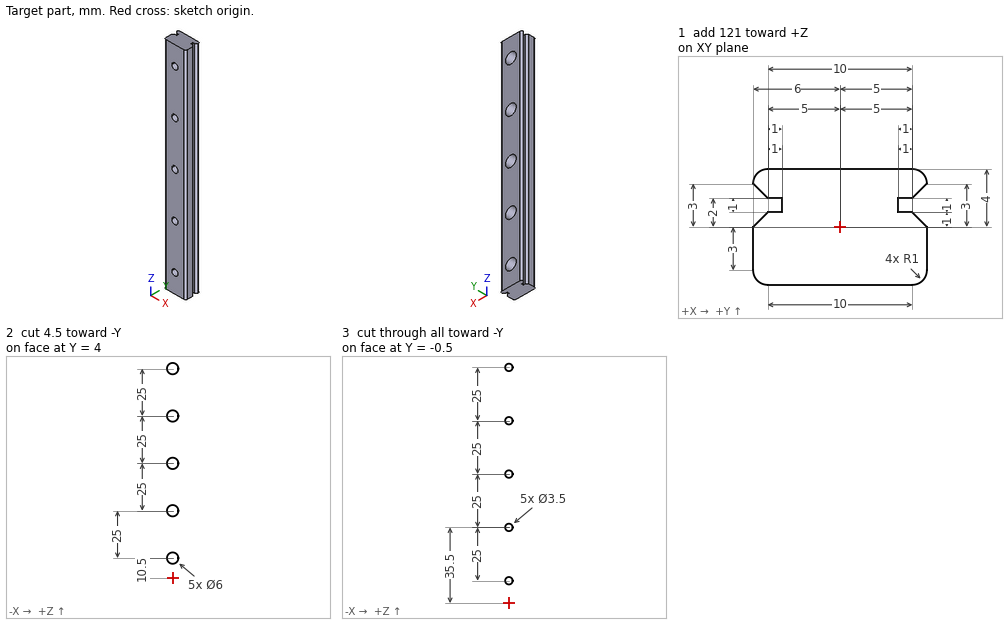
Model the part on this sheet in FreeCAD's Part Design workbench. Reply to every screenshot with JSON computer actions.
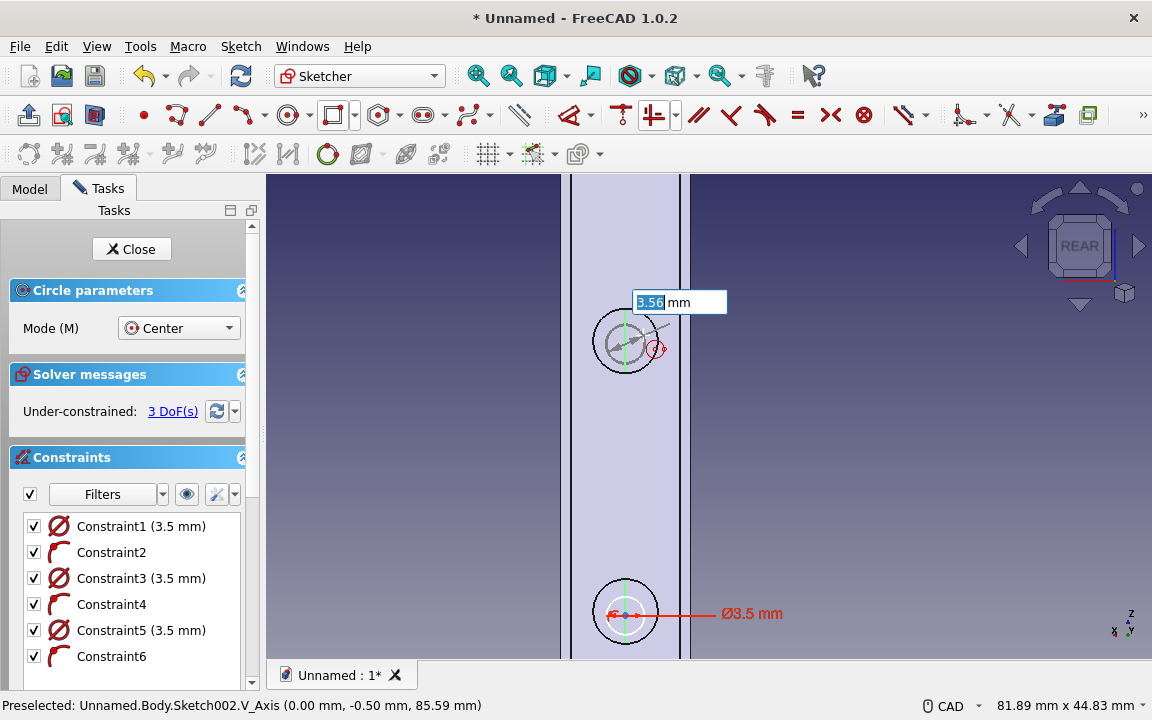
{"action": "type", "text": "3.5"}
{"action": "key", "text": "Return"}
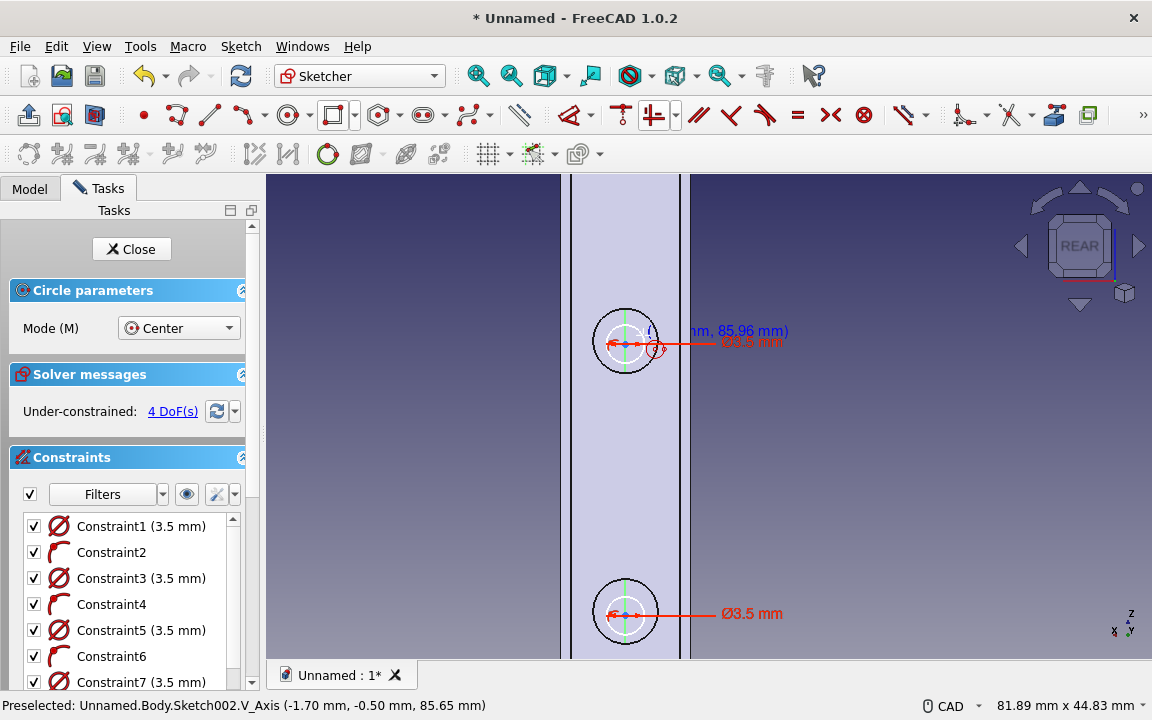
{"action": "scroll", "coordinate": [645, 337], "scroll_direction": "down", "scroll_amount": 7}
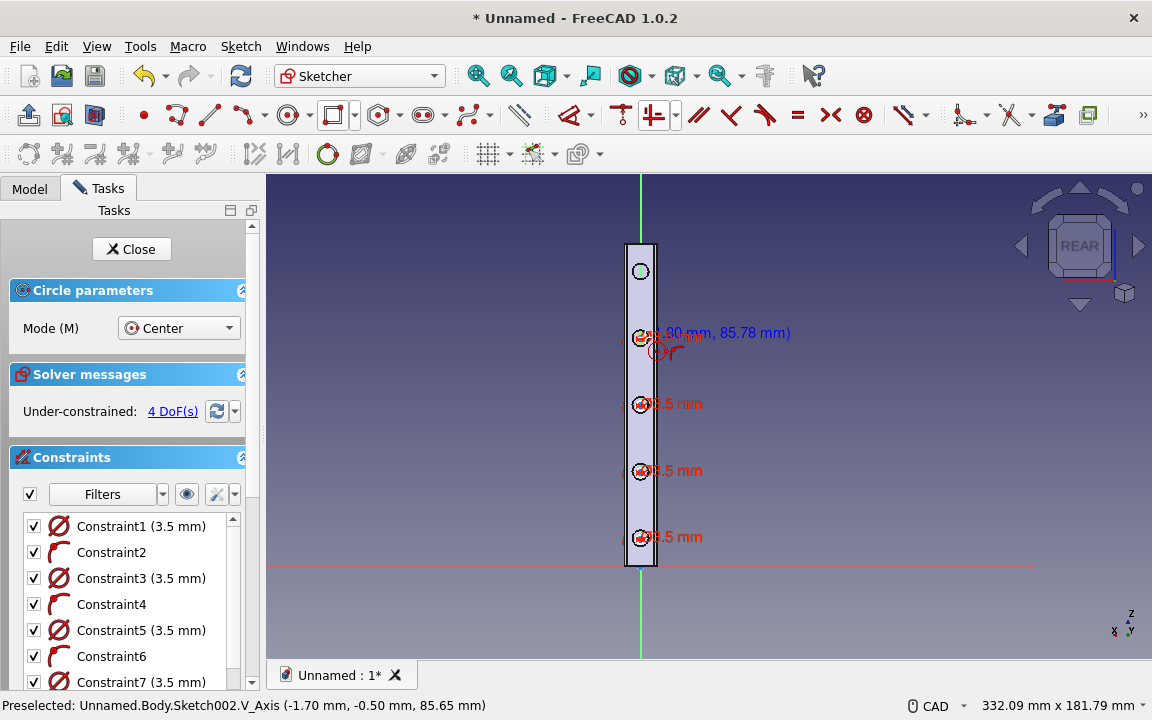
{"action": "scroll", "coordinate": [641, 272], "scroll_direction": "up", "scroll_amount": 8}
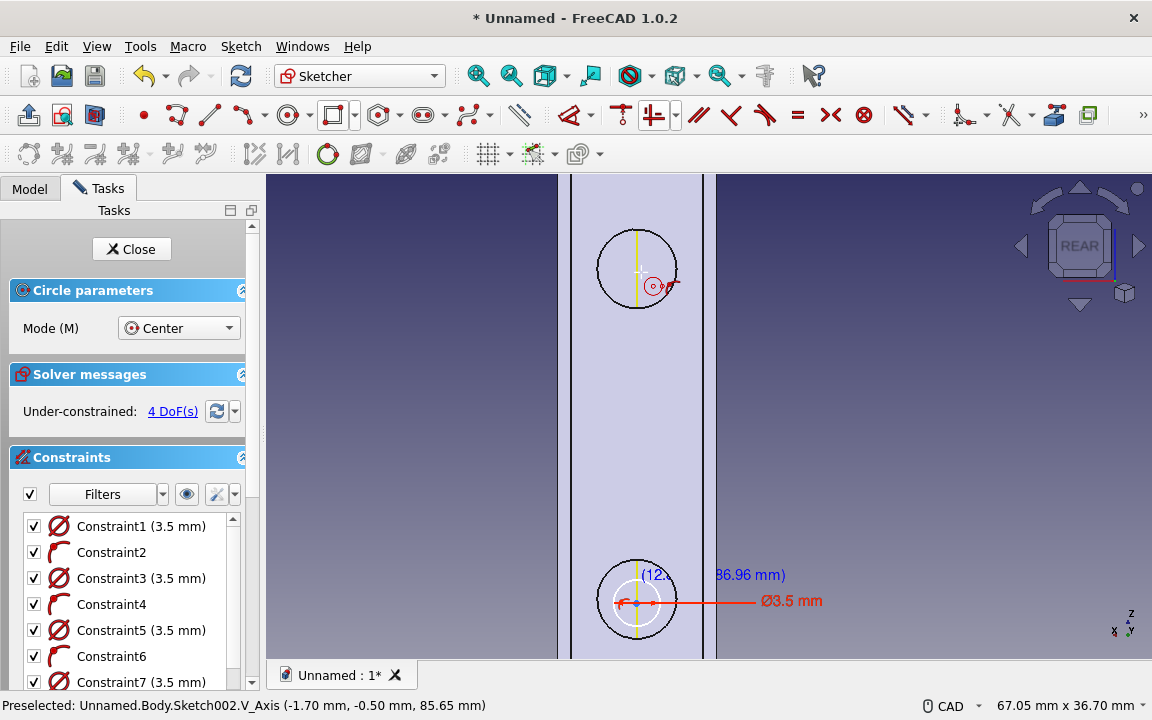
{"action": "scroll", "coordinate": [641, 272], "scroll_direction": "down", "scroll_amount": 8}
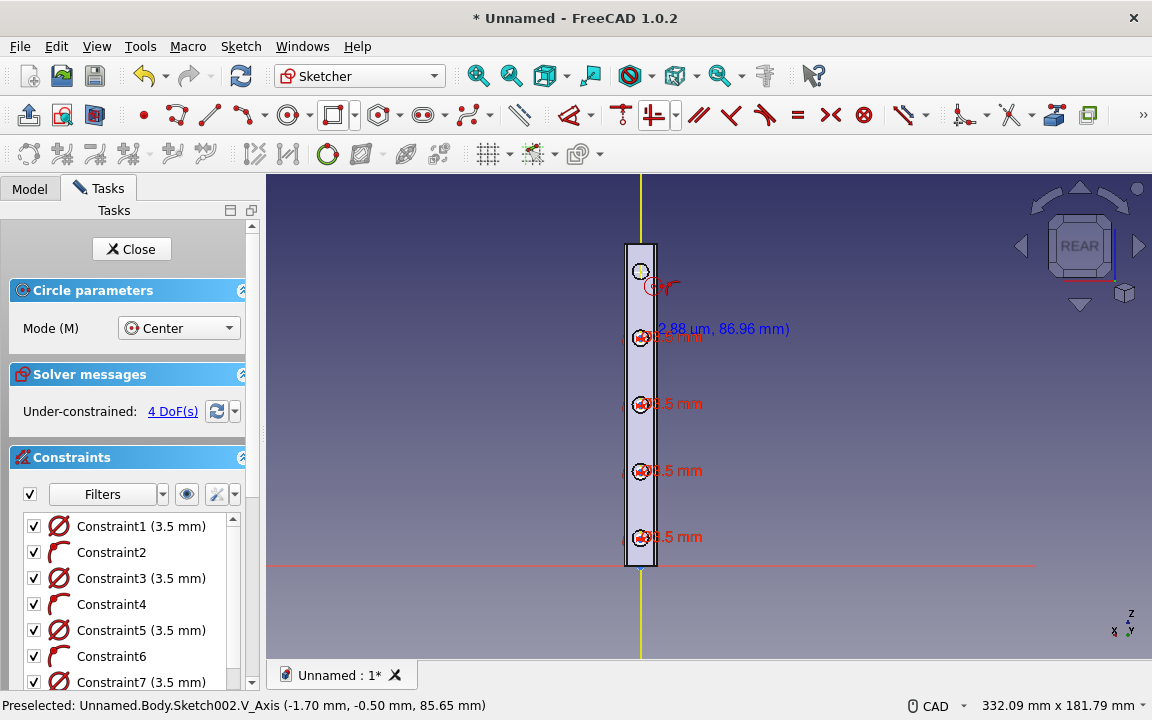
{"action": "left_click", "coordinate": [641, 272]}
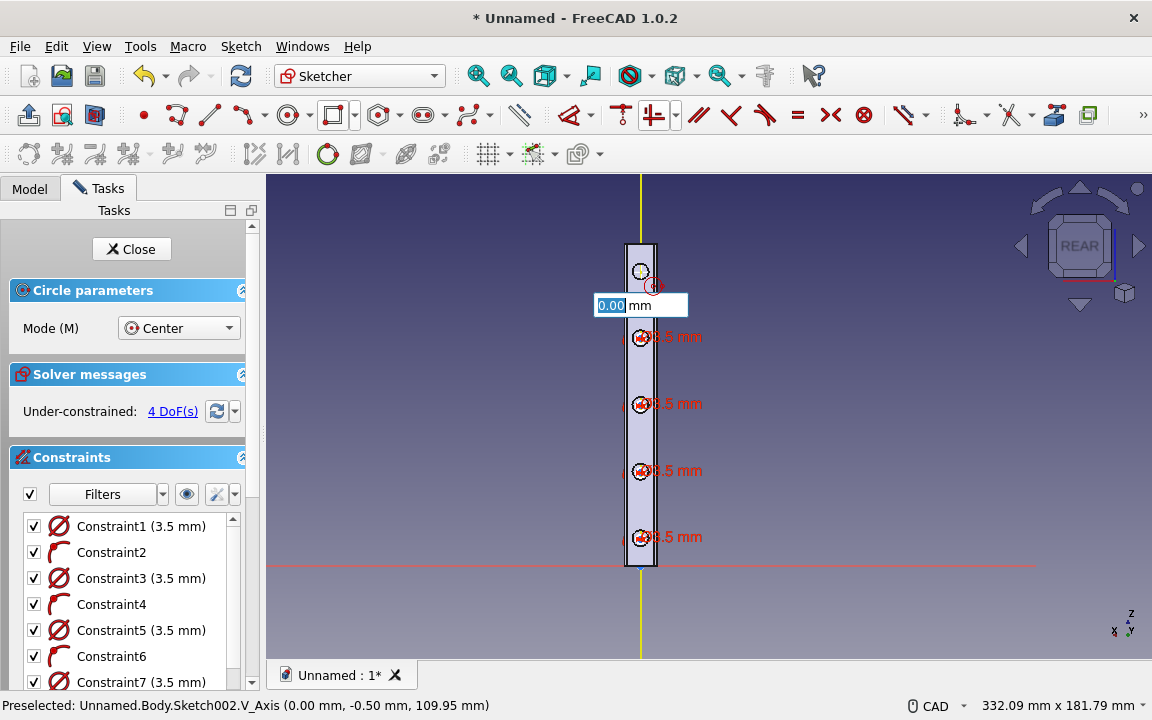
{"action": "scroll", "coordinate": [645, 270], "scroll_direction": "up", "scroll_amount": 7}
{"action": "mouse_move", "coordinate": [643, 269]}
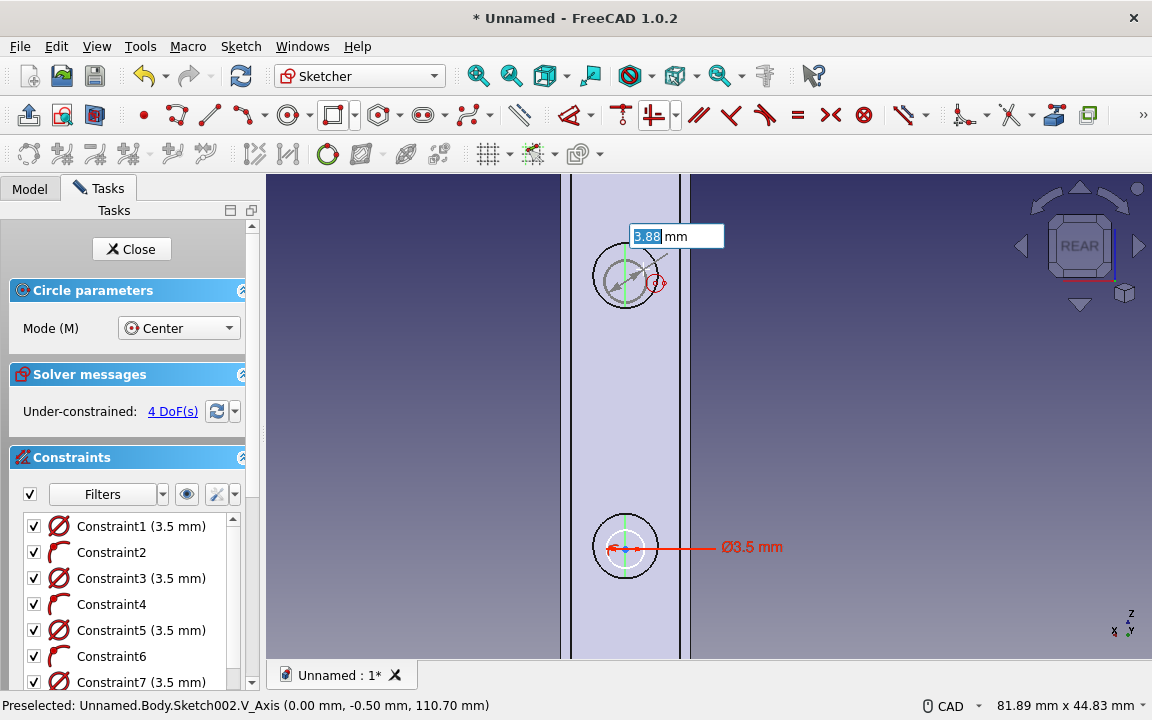
{"action": "type", "text": "3.5"}
{"action": "key", "text": "Return"}
{"action": "key", "text": "Escape"}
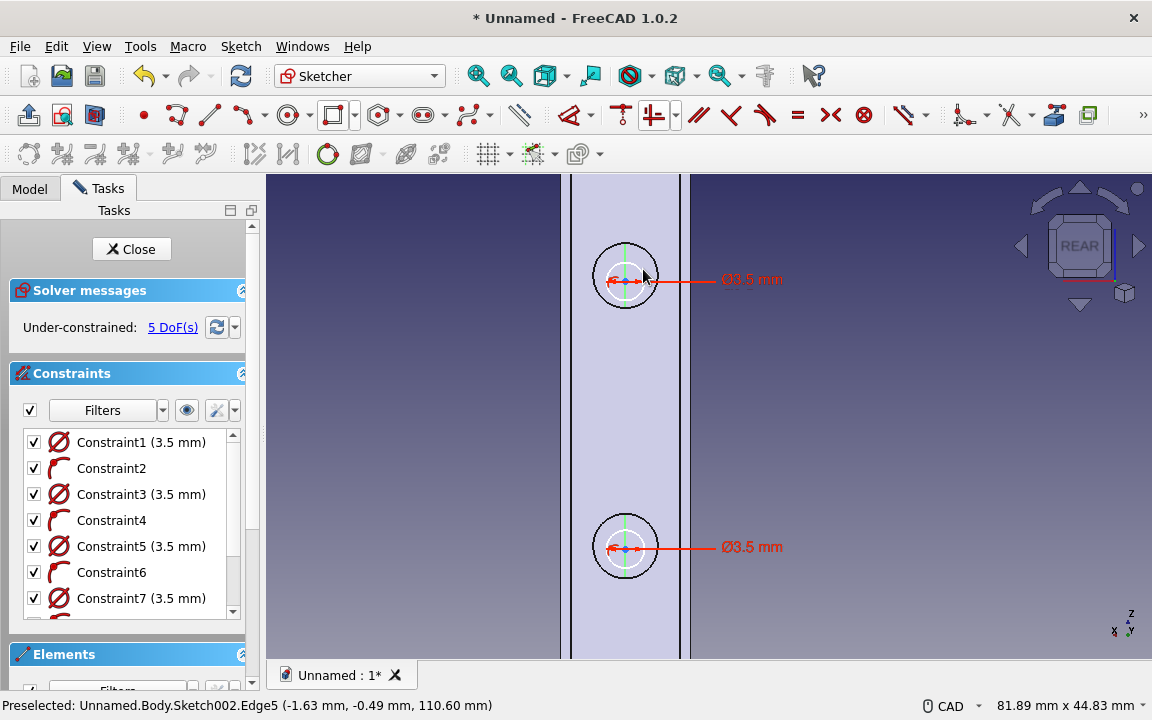
{"action": "left_click", "coordinate": [568, 116]}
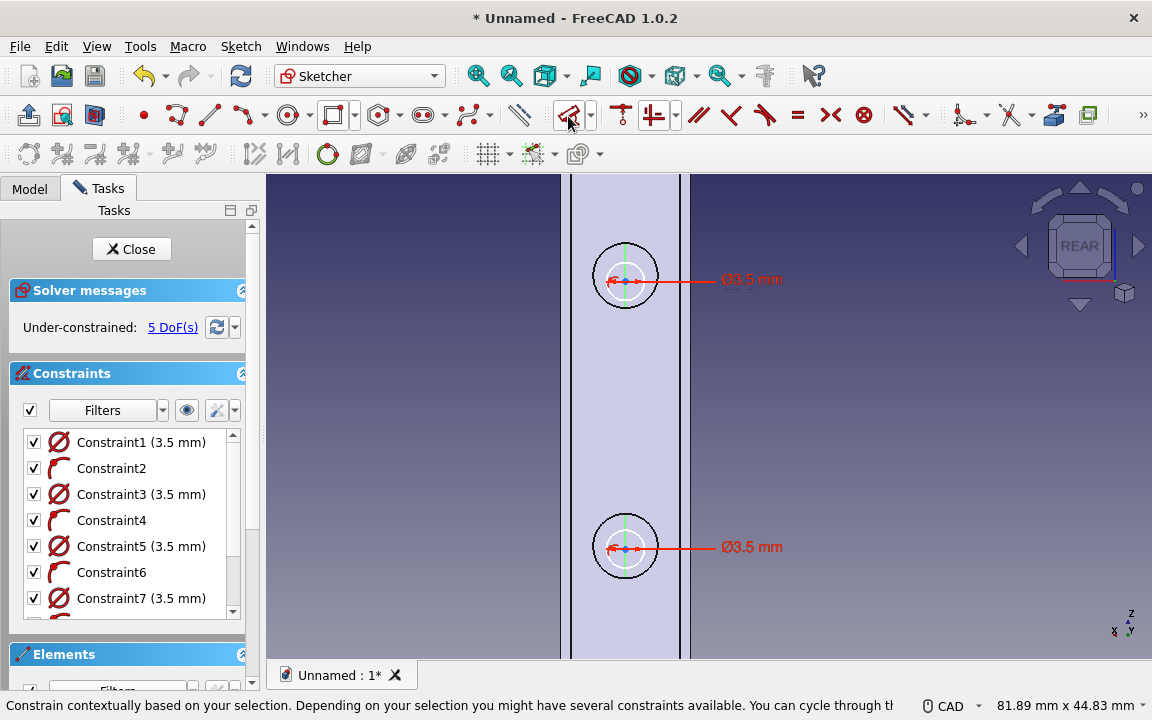
{"action": "scroll", "coordinate": [645, 270], "scroll_direction": "down", "scroll_amount": 7}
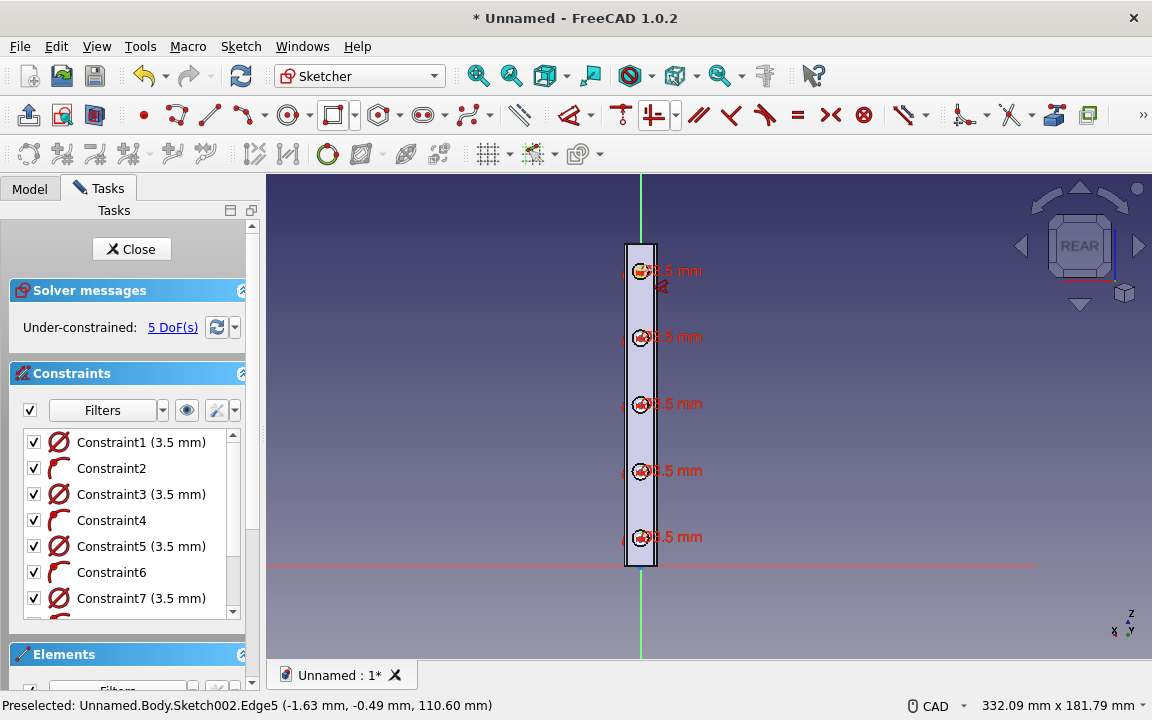
{"action": "left_click", "coordinate": [641, 473]}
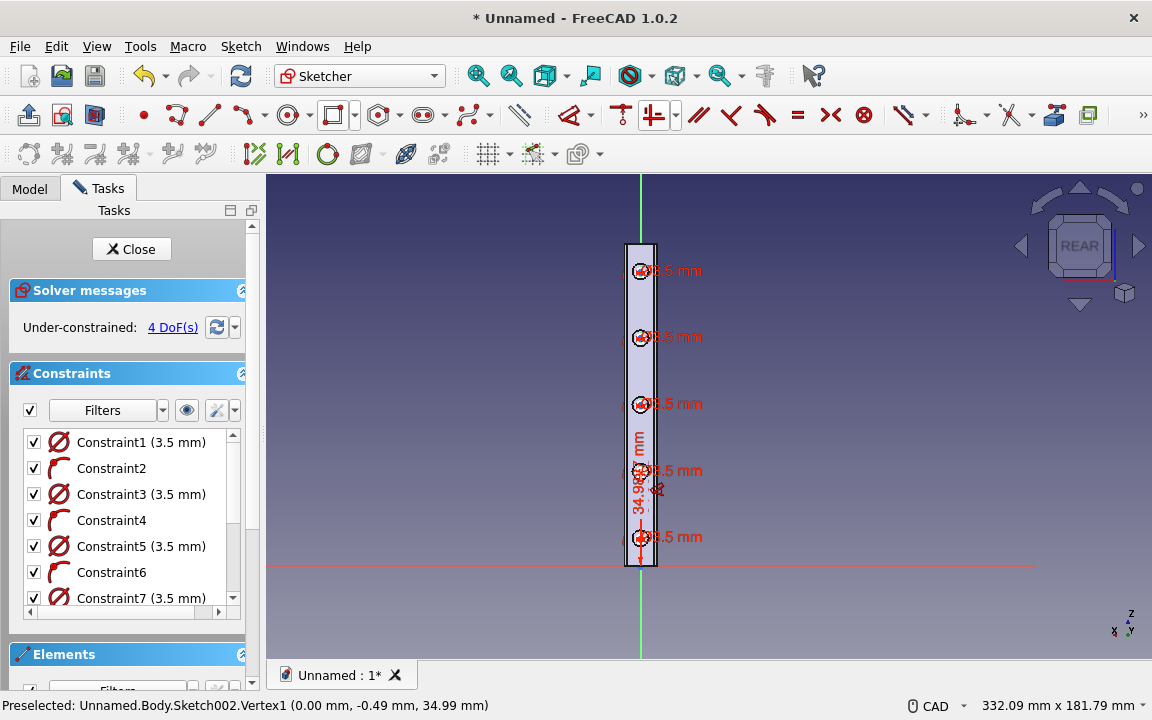
{"action": "left_click", "coordinate": [641, 539]}
{"action": "left_click", "coordinate": [675, 506]}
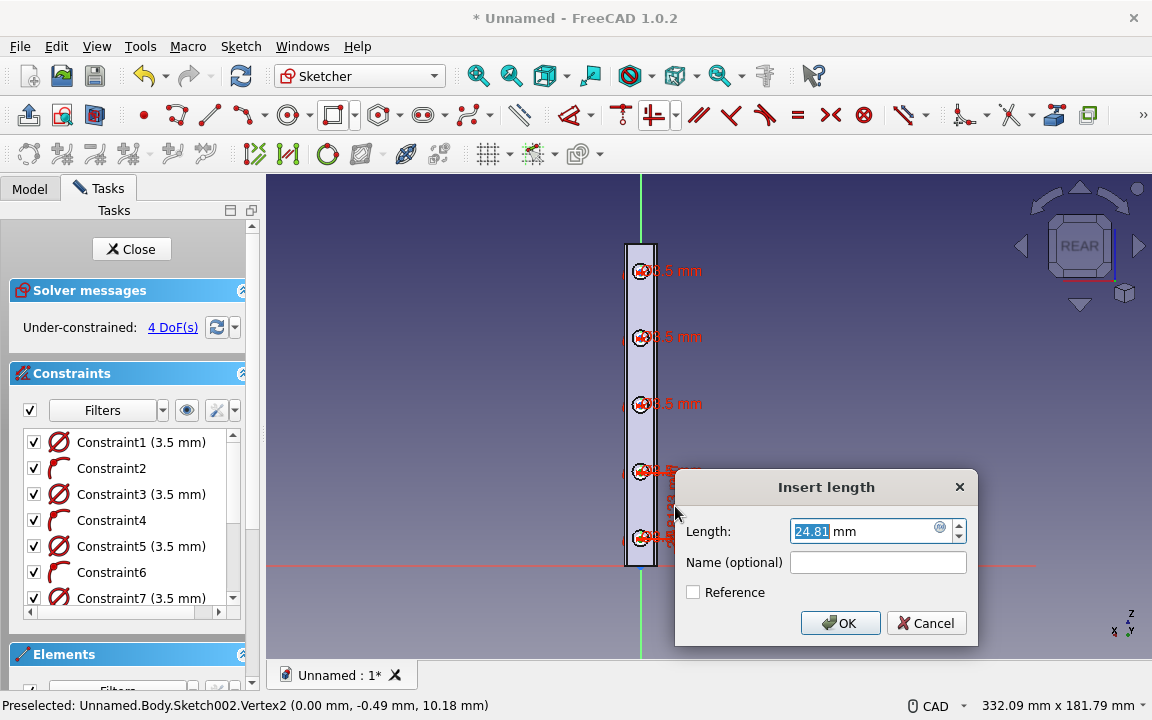
{"action": "type", "text": "25"}
{"action": "key", "text": "Return"}